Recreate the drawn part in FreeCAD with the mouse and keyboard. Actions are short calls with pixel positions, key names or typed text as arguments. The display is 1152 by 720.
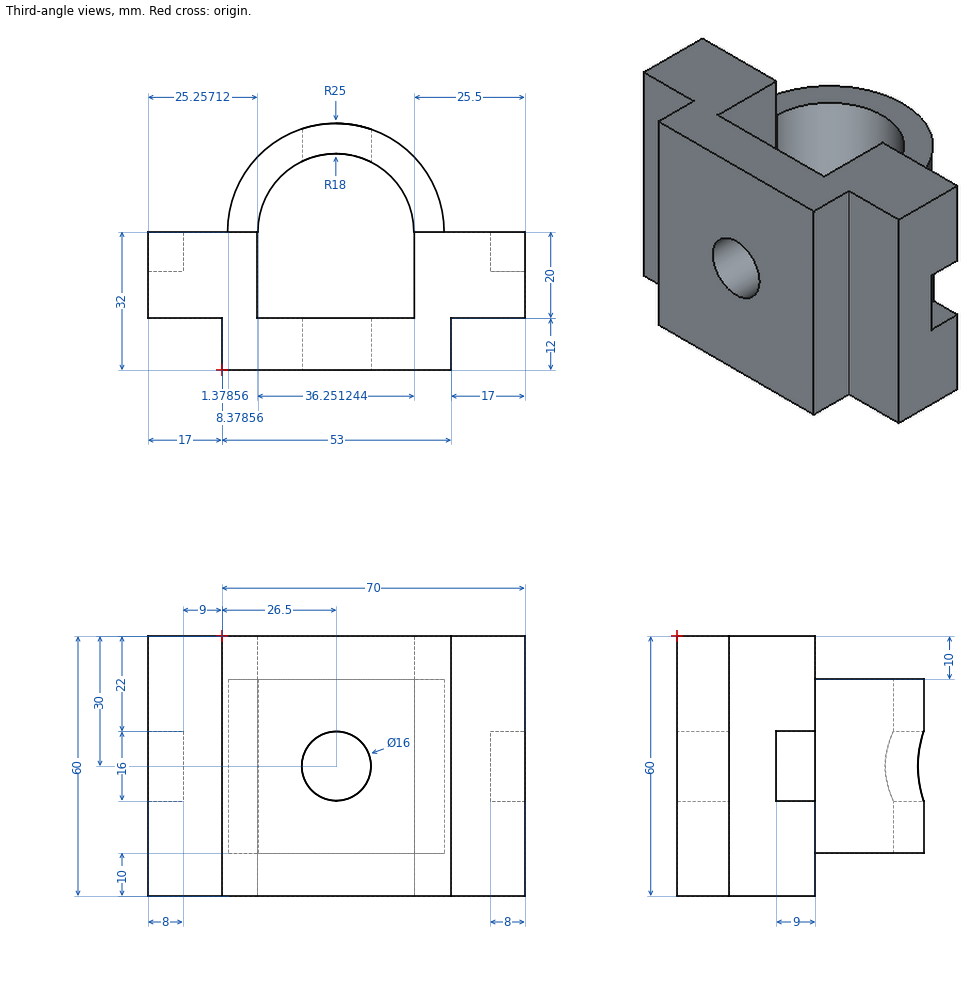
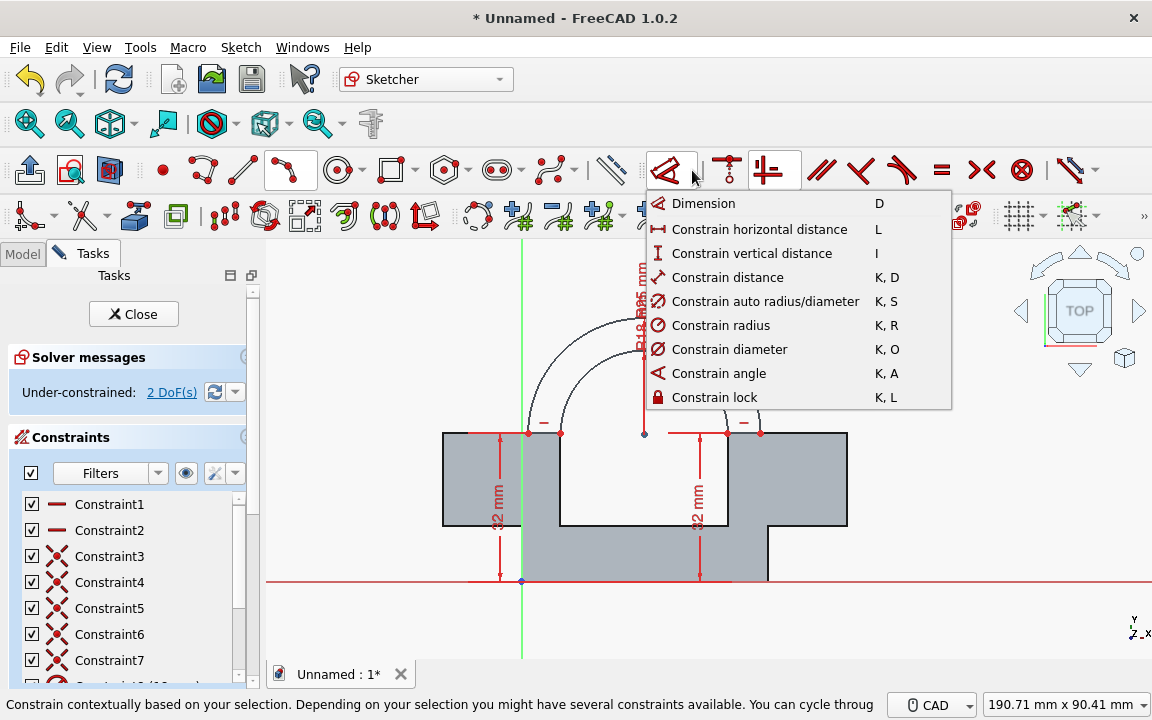
click(799, 253)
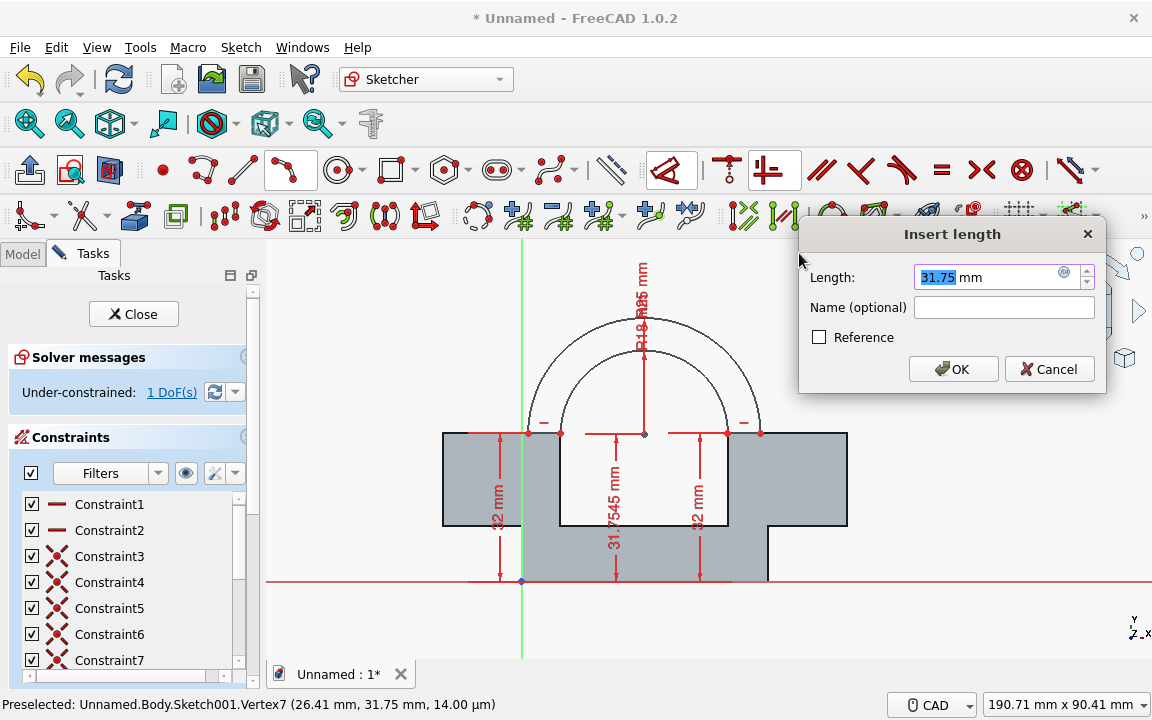
text(32)
key(Return)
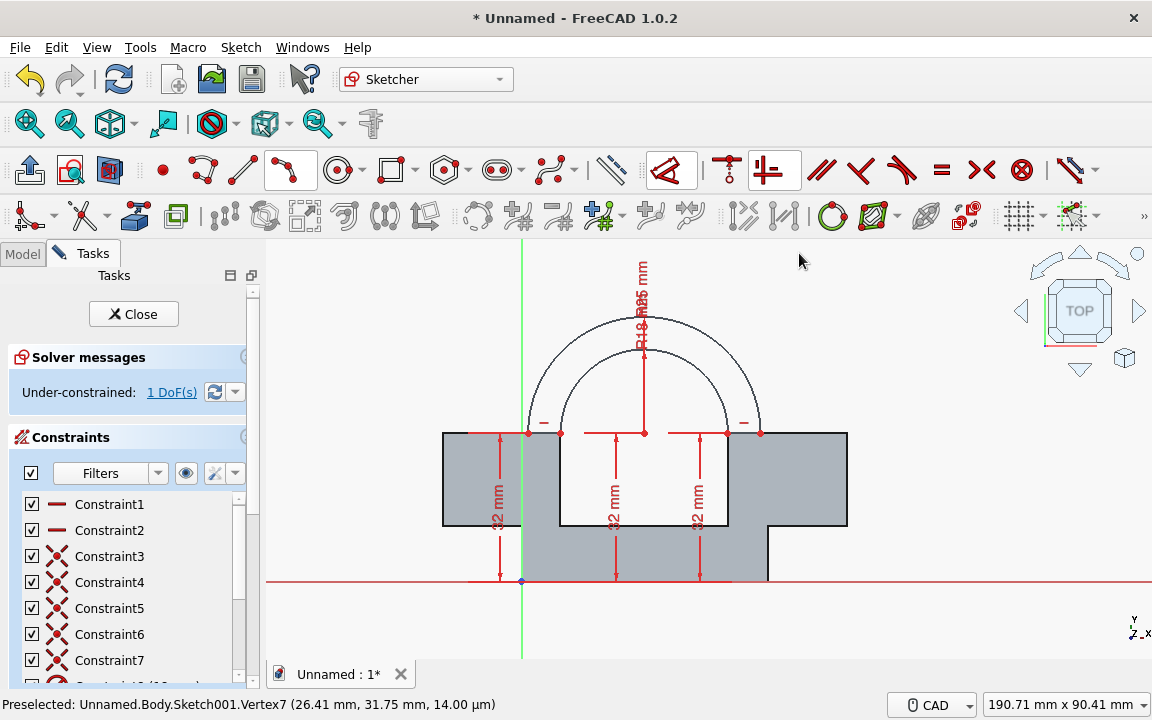
scroll(528, 433, up, 10)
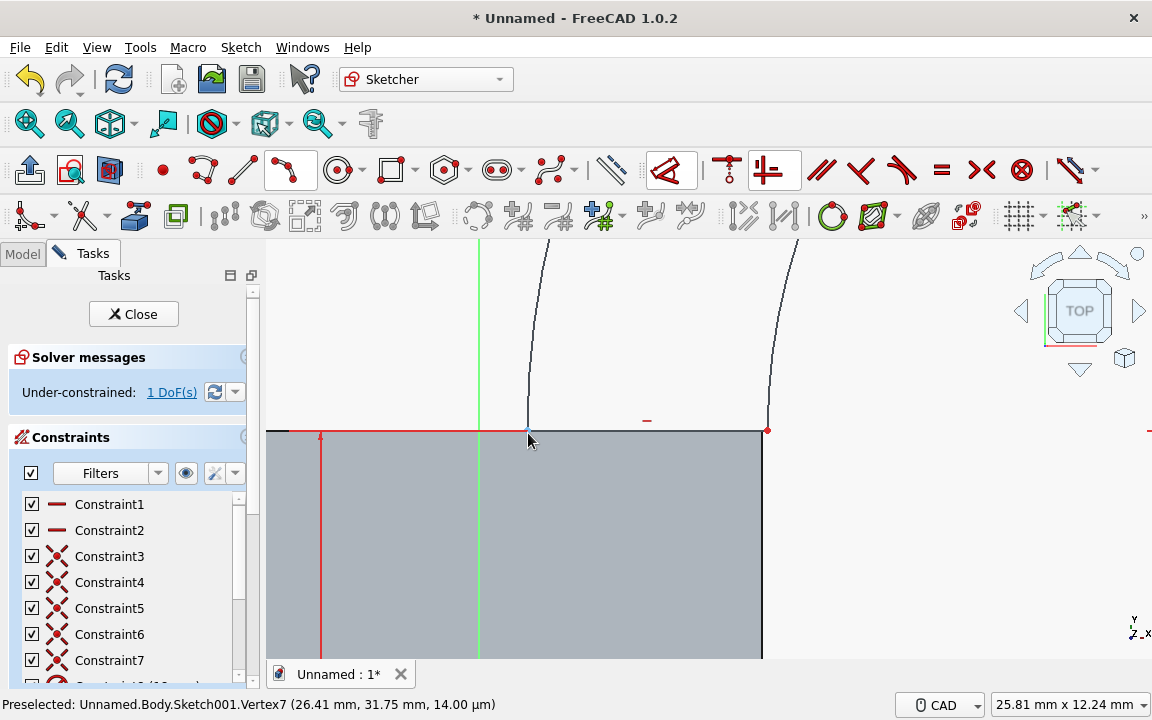
click(527, 431)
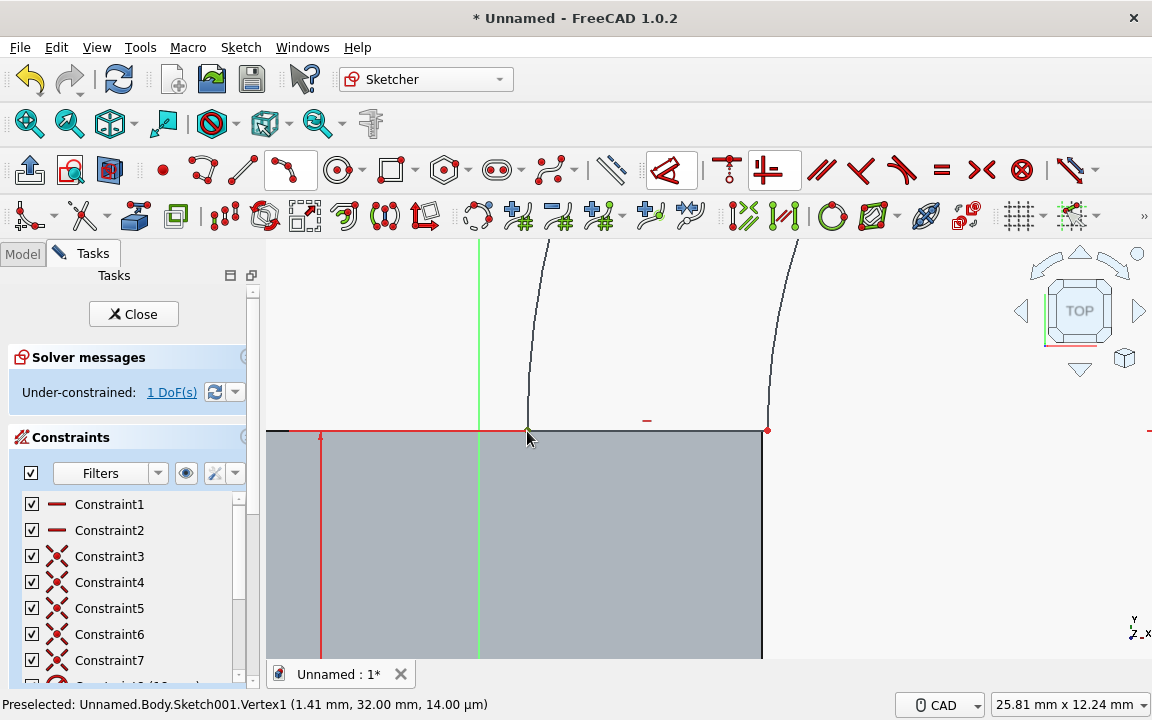
key(l)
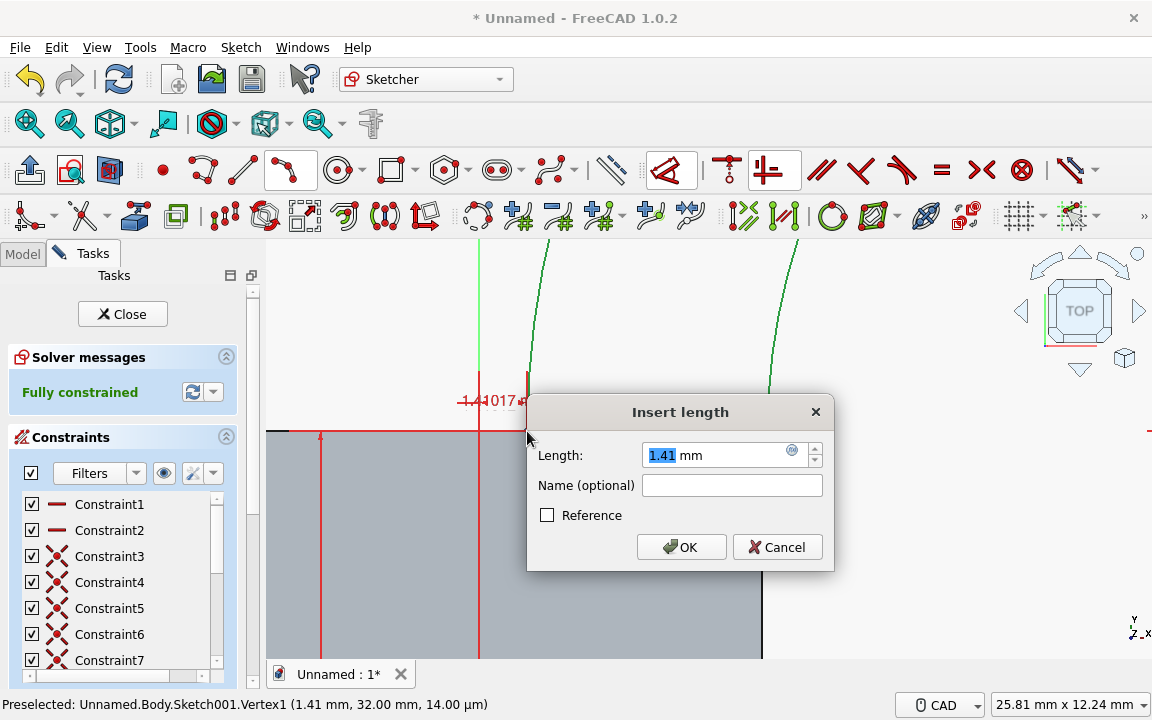
text(1.37856)
key(Return)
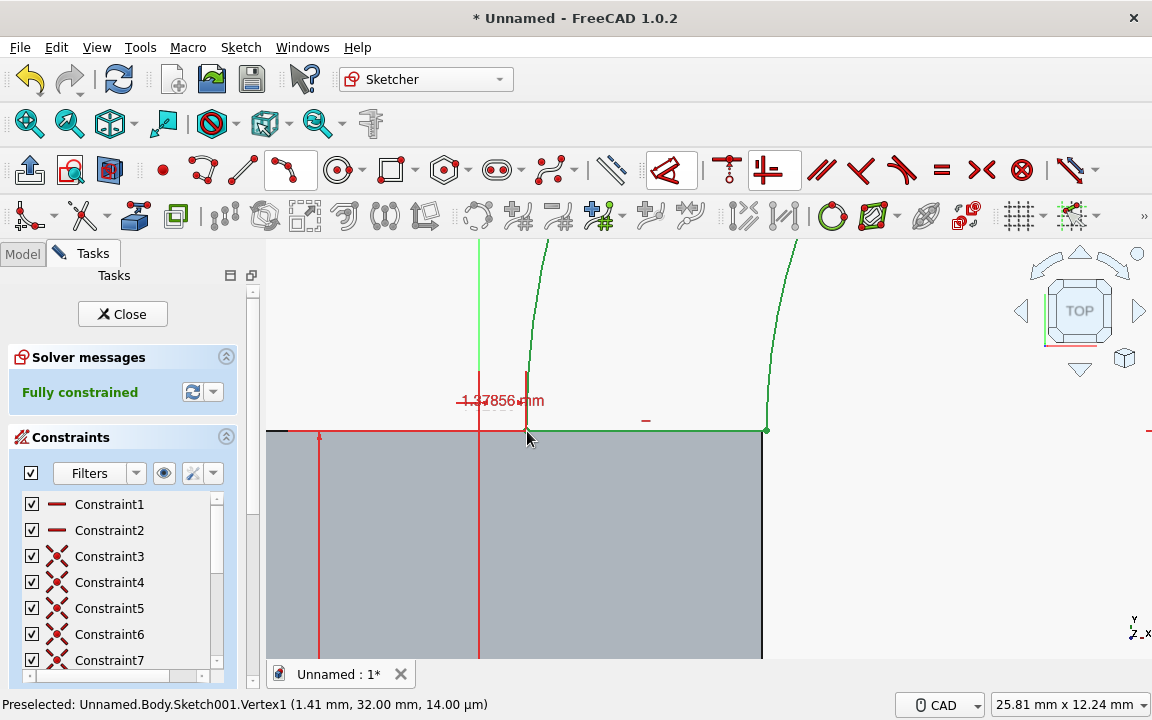
click(123, 314)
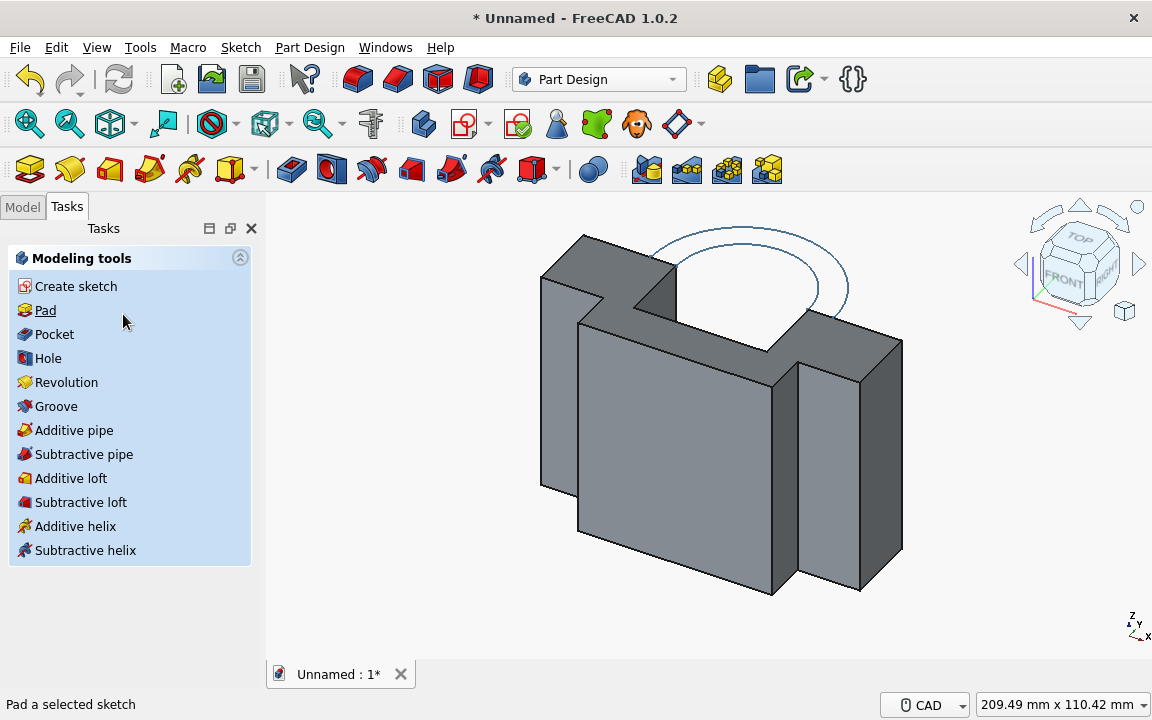
click(30, 170)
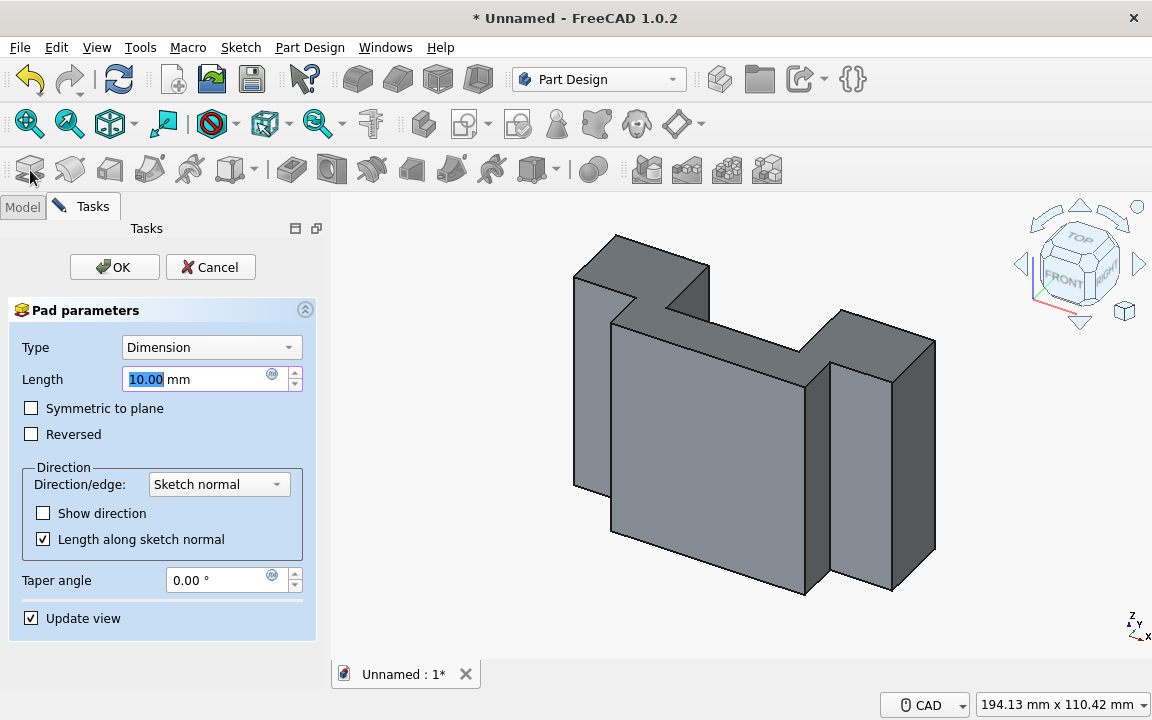
text(60)
key(Tab)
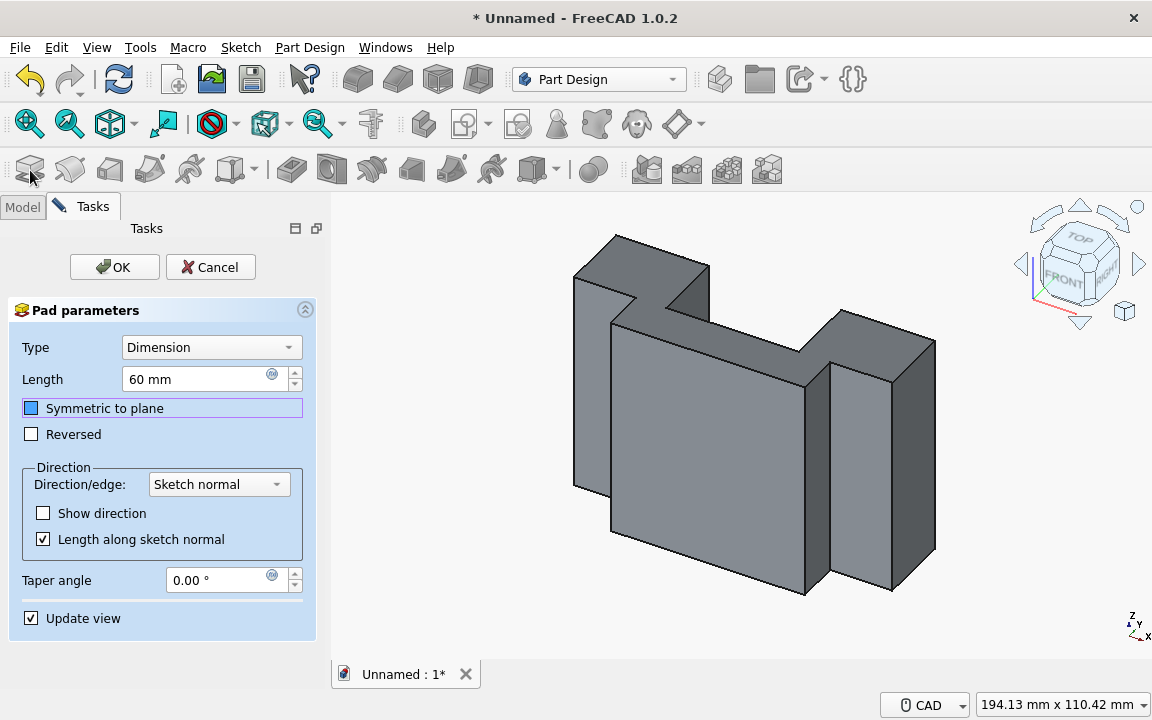
click(30, 434)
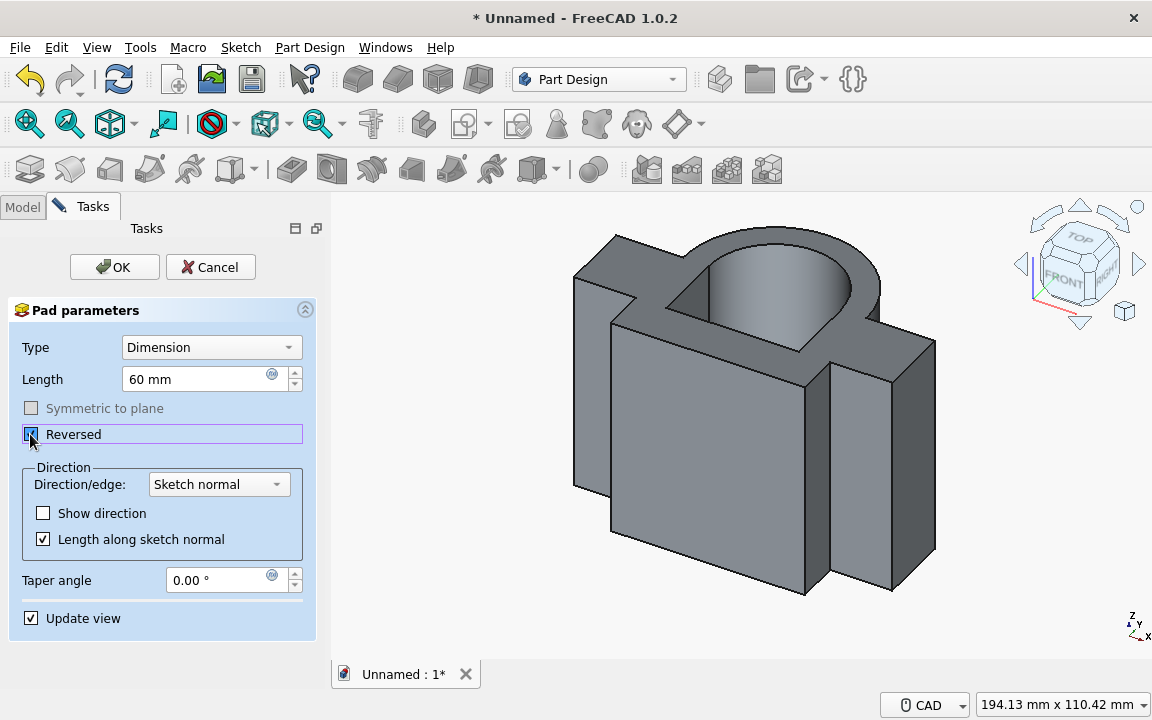
click(115, 267)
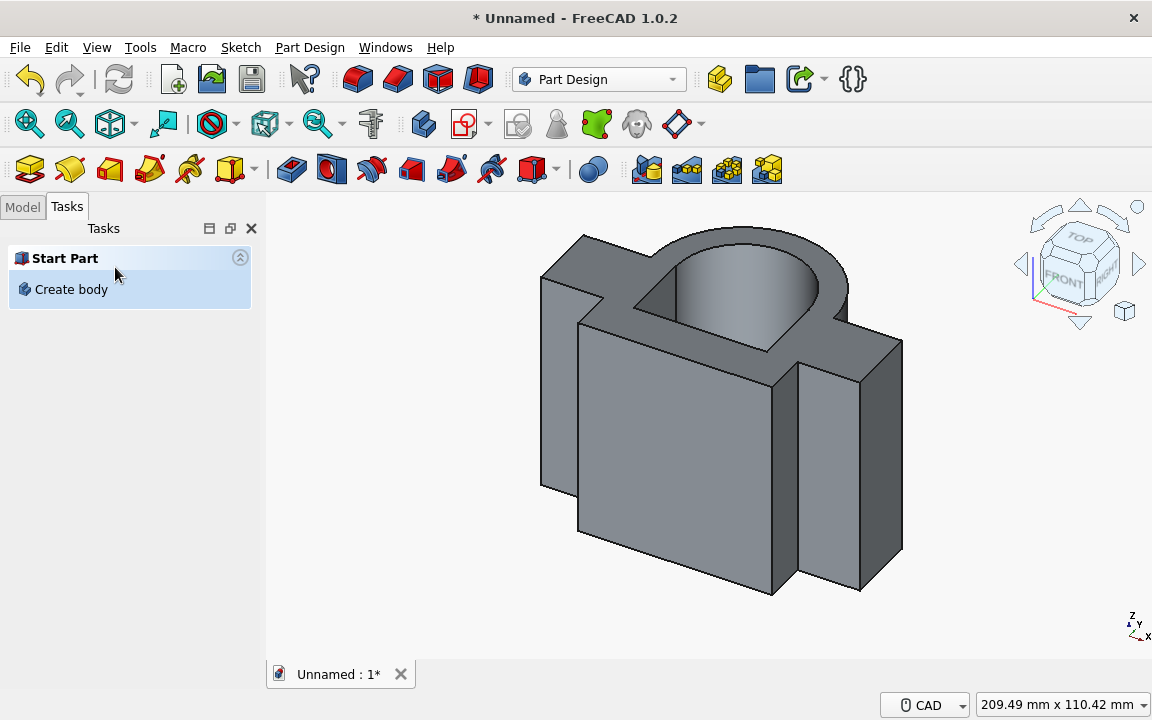
click(30, 124)